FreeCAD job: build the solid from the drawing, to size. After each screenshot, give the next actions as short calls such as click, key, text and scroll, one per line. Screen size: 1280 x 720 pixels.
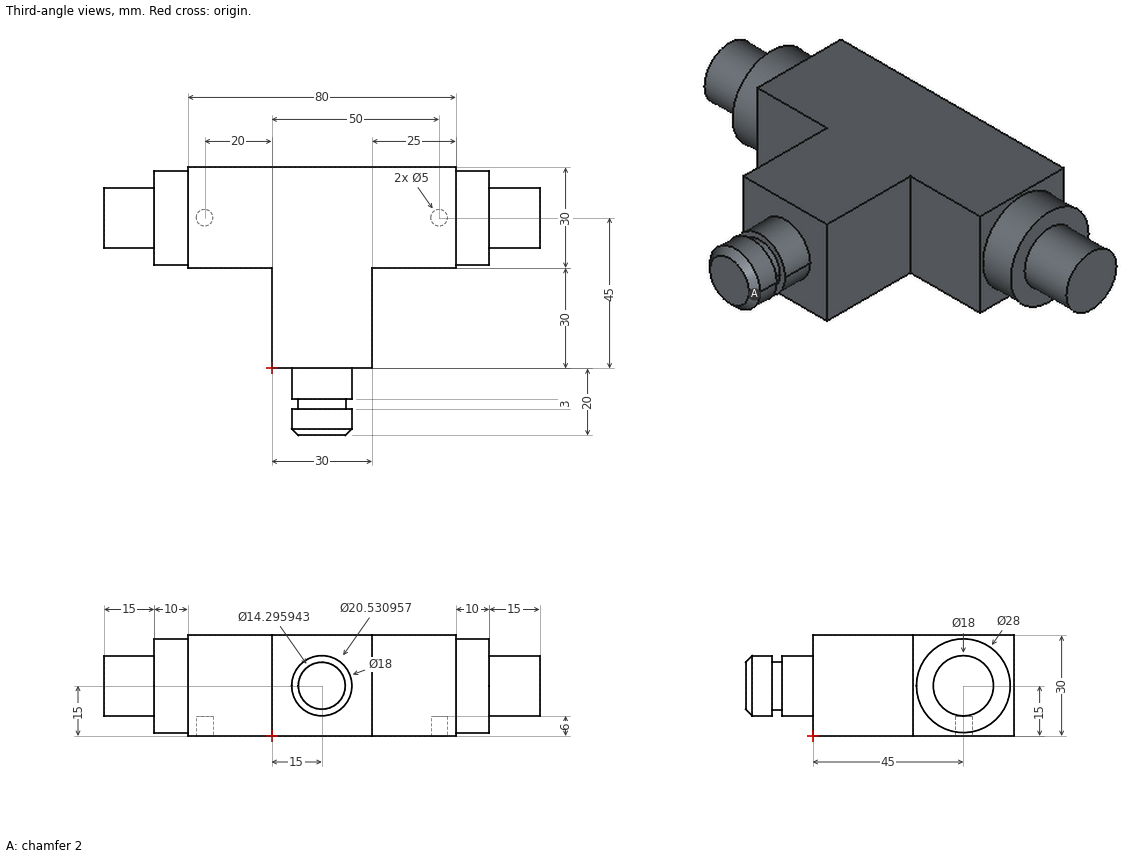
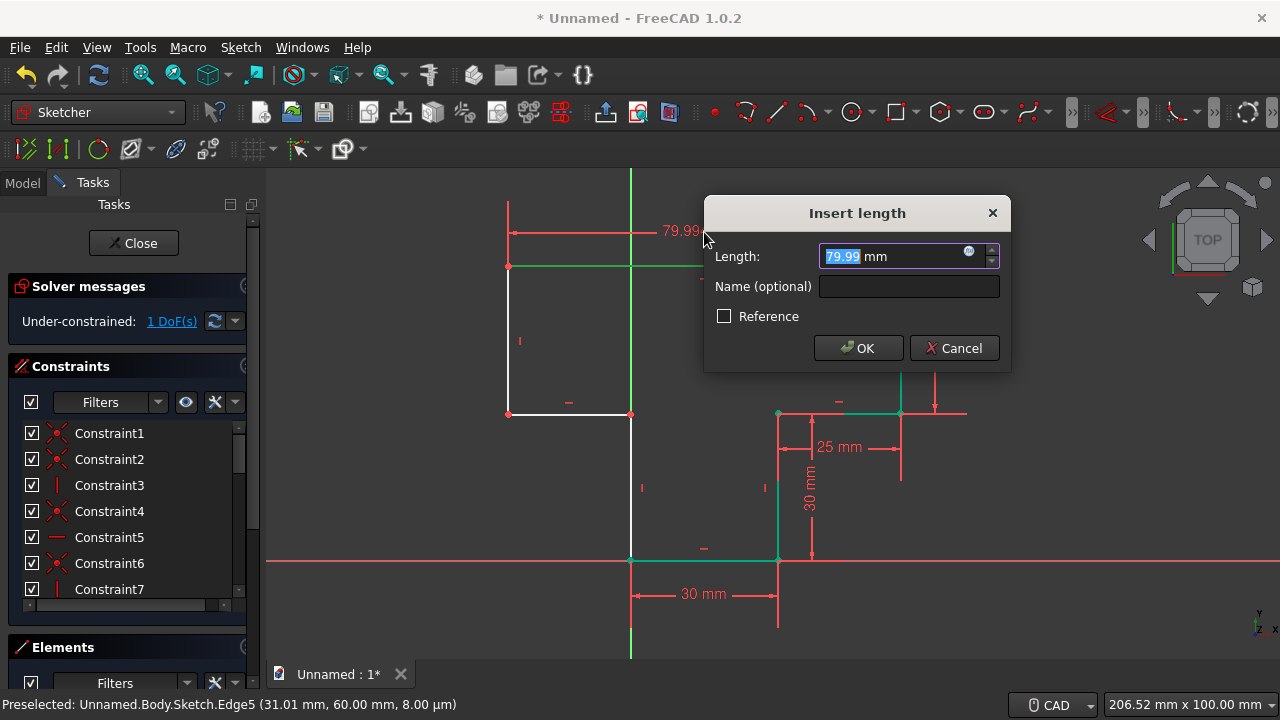
text(80)
key(Return)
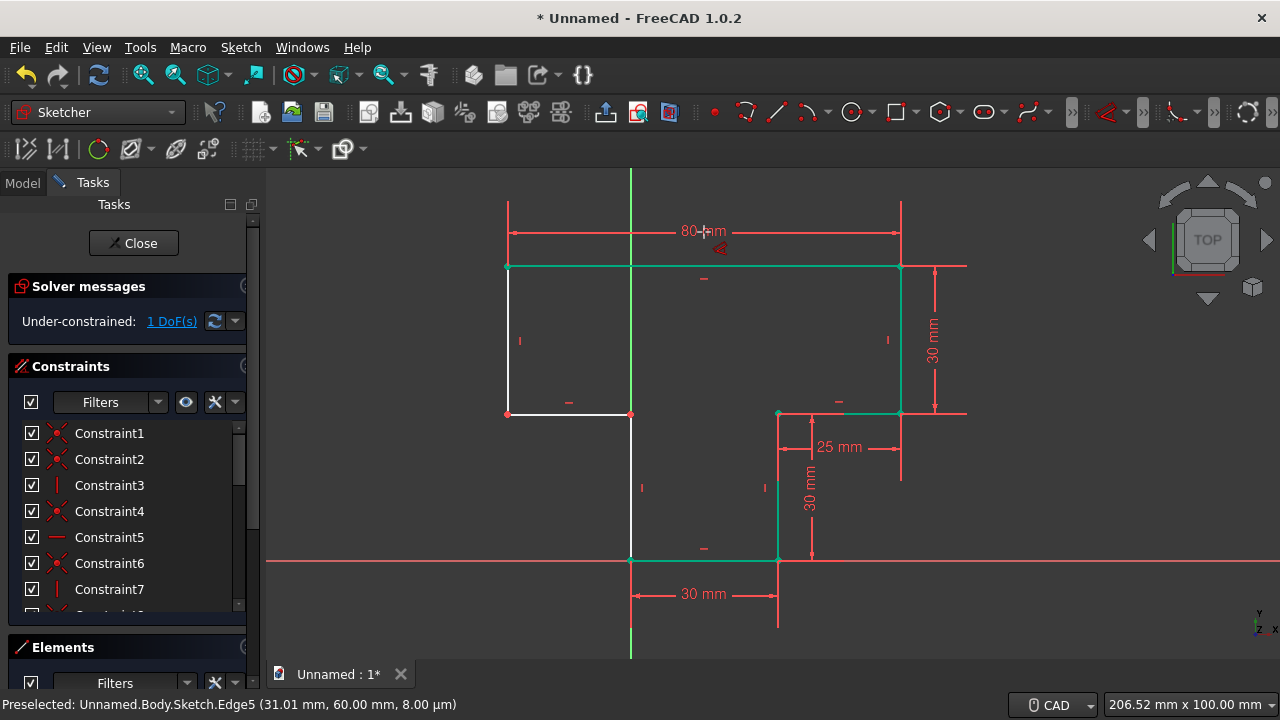
click(508, 311)
click(474, 341)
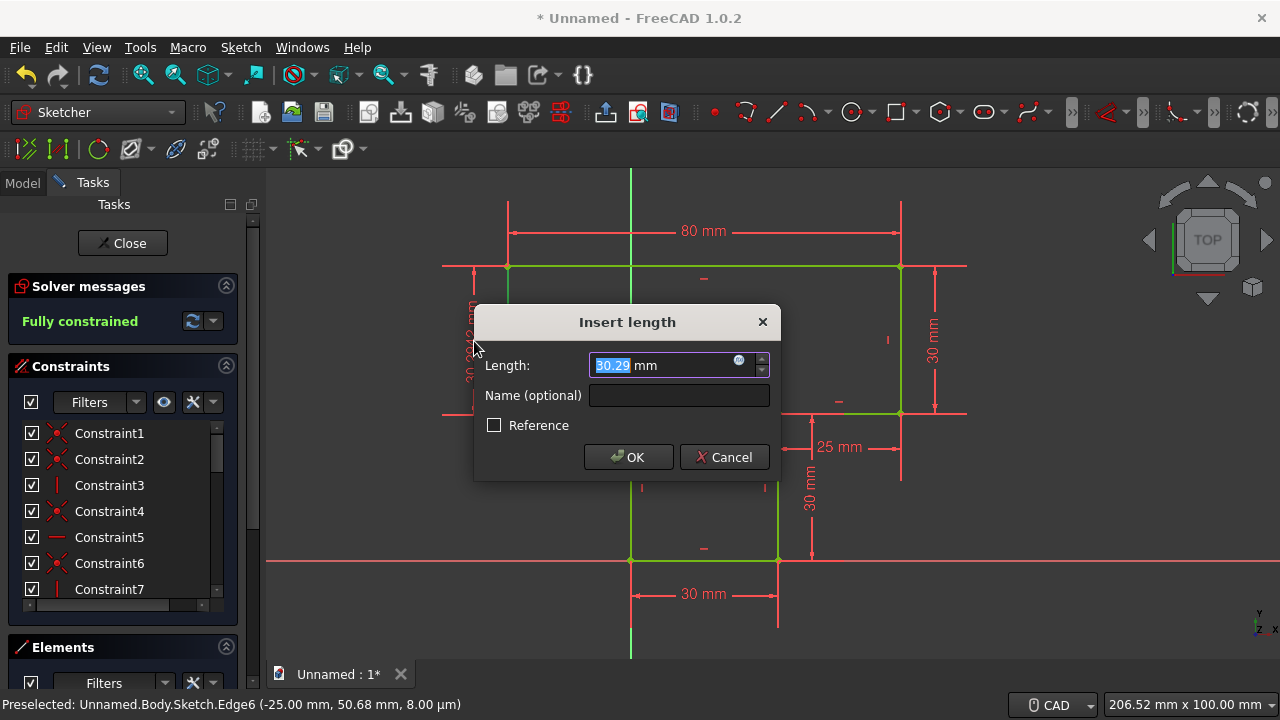
text(30)
key(Return)
key(Escape)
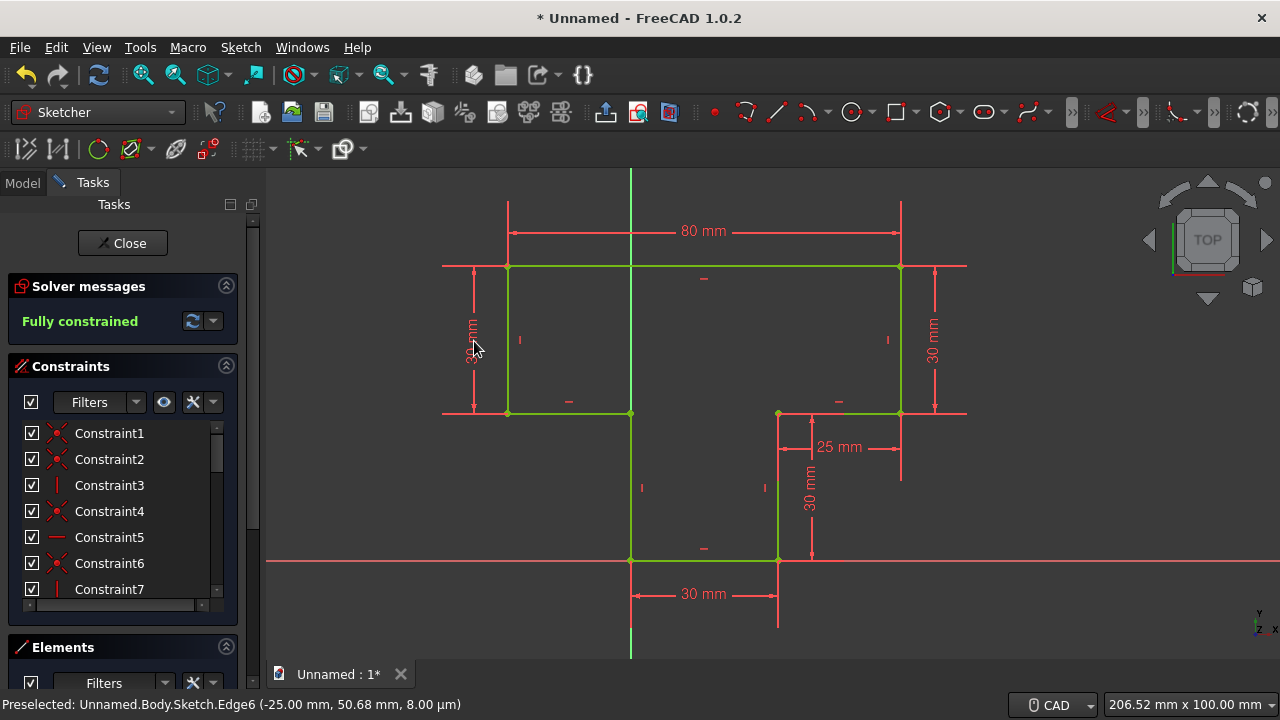
click(123, 243)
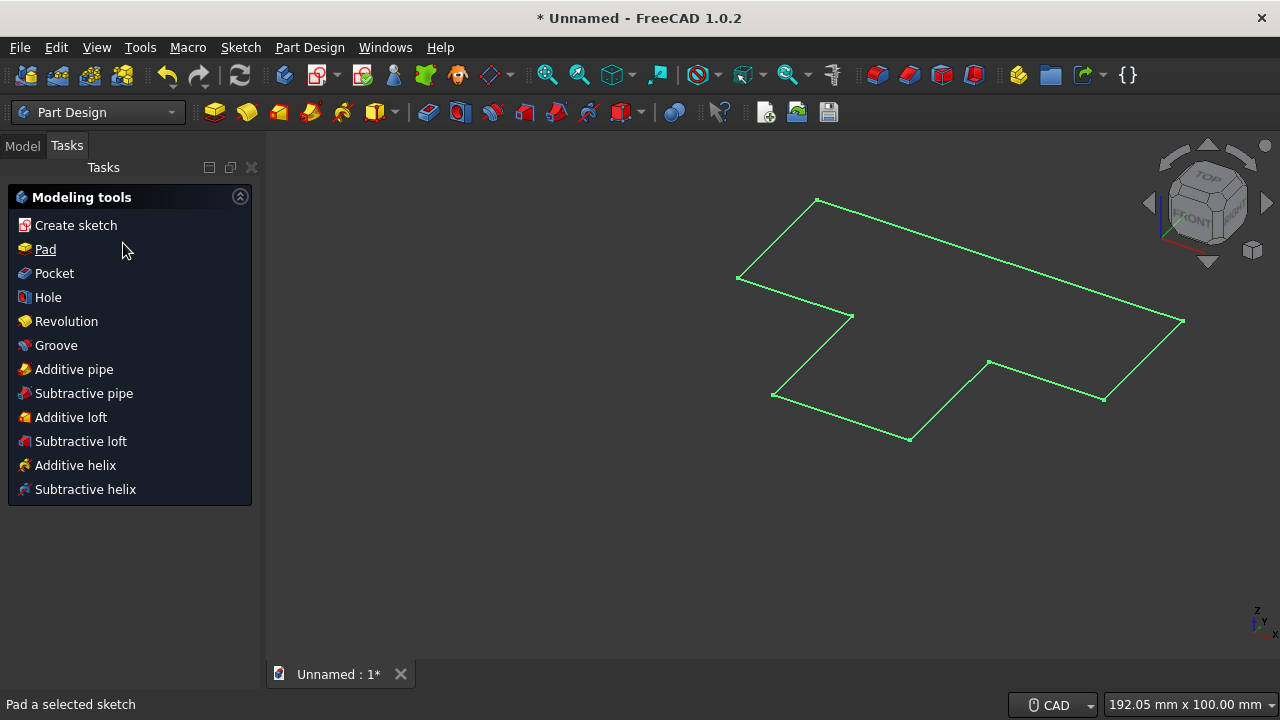
click(216, 112)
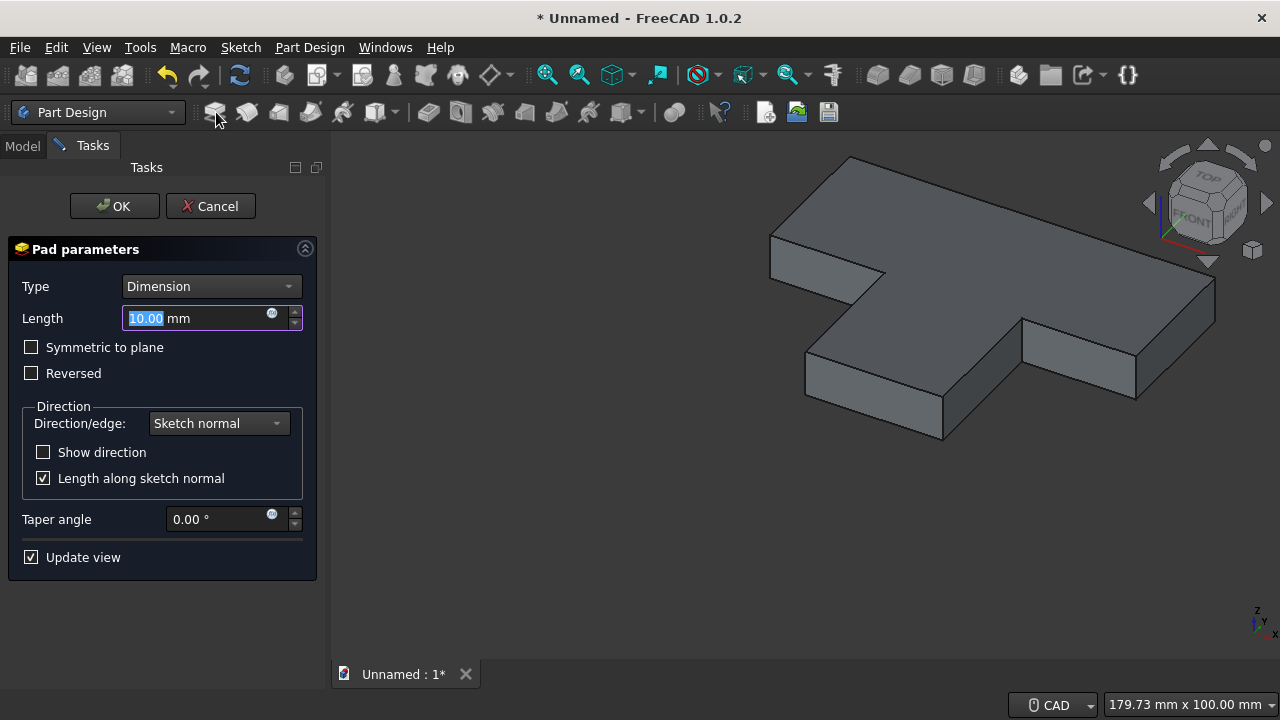
text(30)
key(Tab)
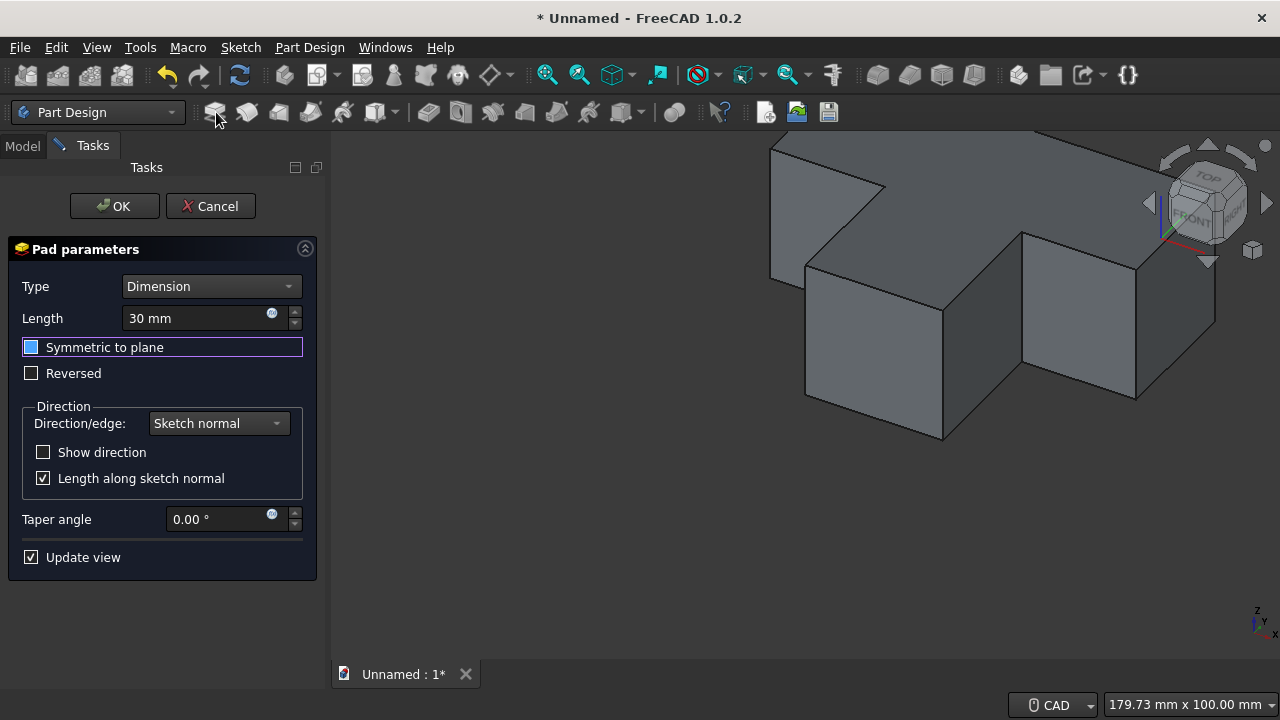
click(115, 206)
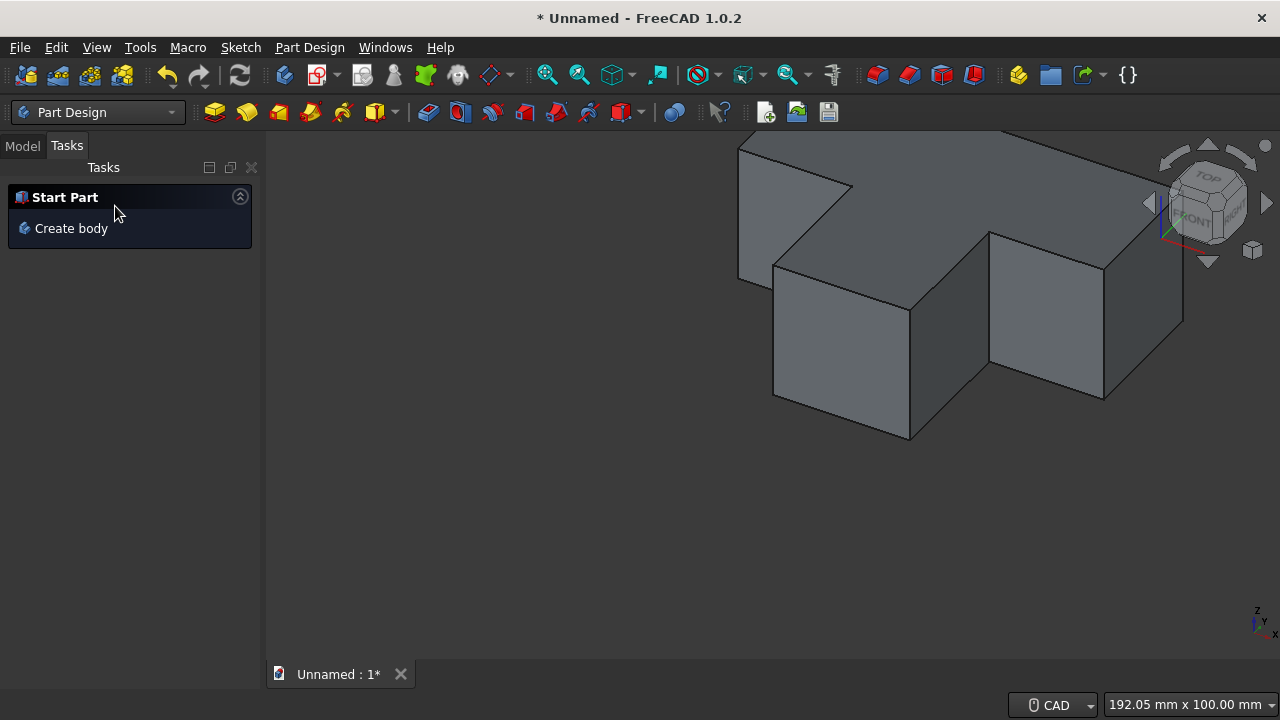
key(v)
key(f)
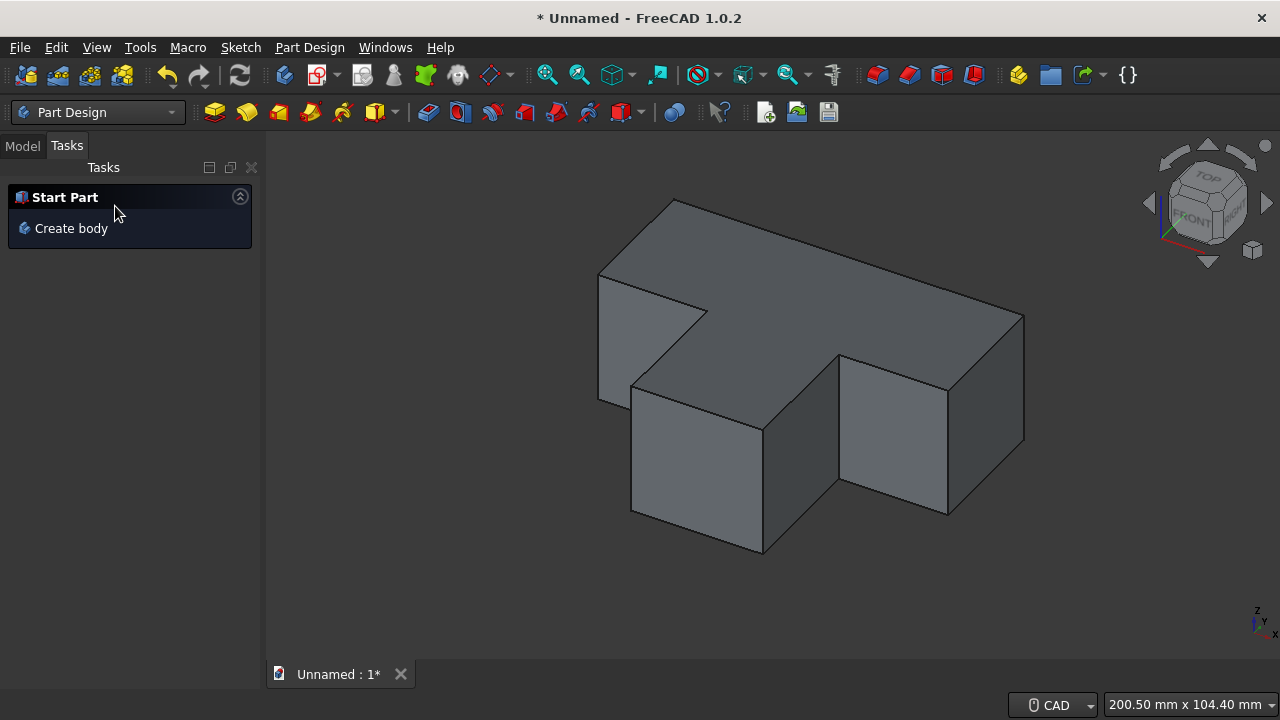
click(986, 414)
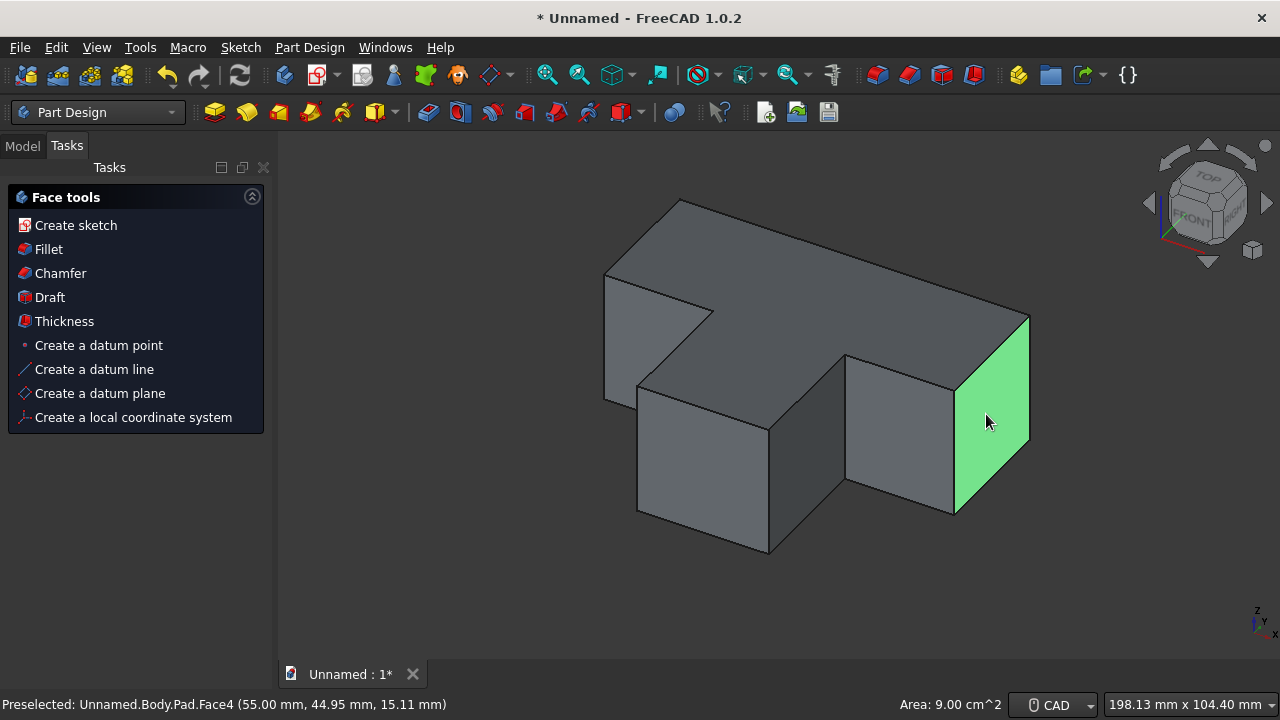
click(318, 76)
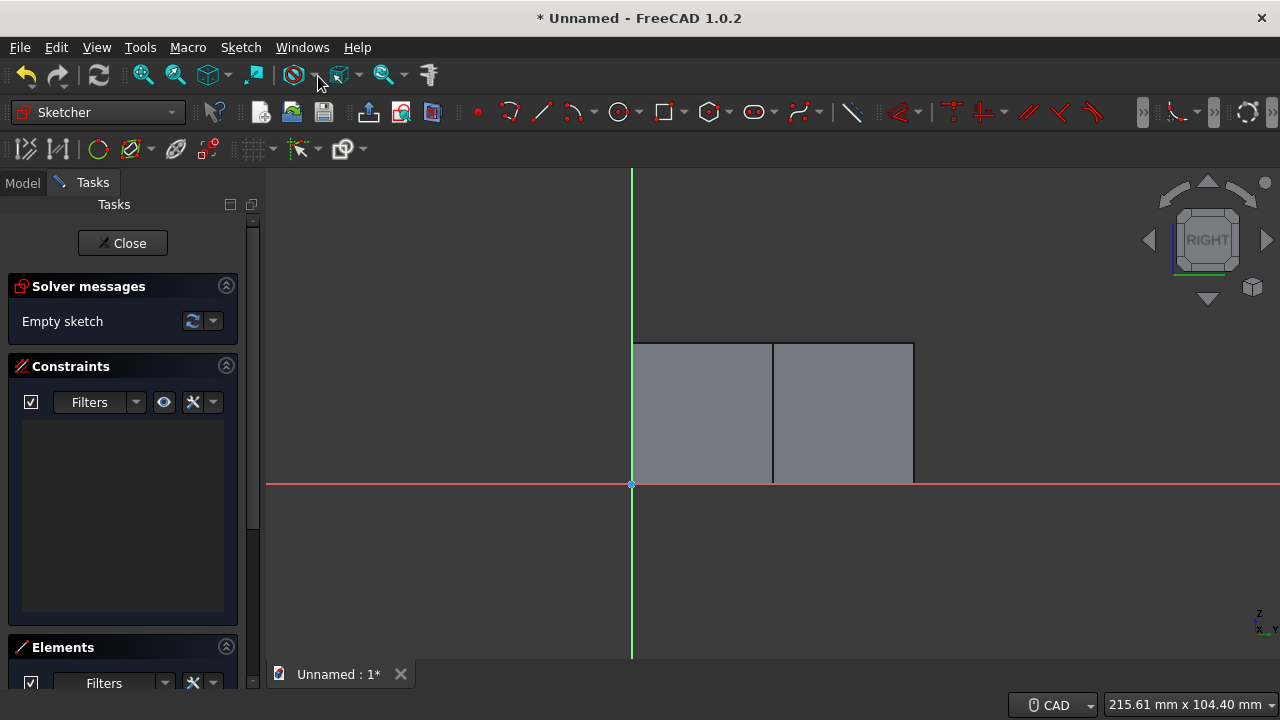
scroll(825, 418, up, 4)